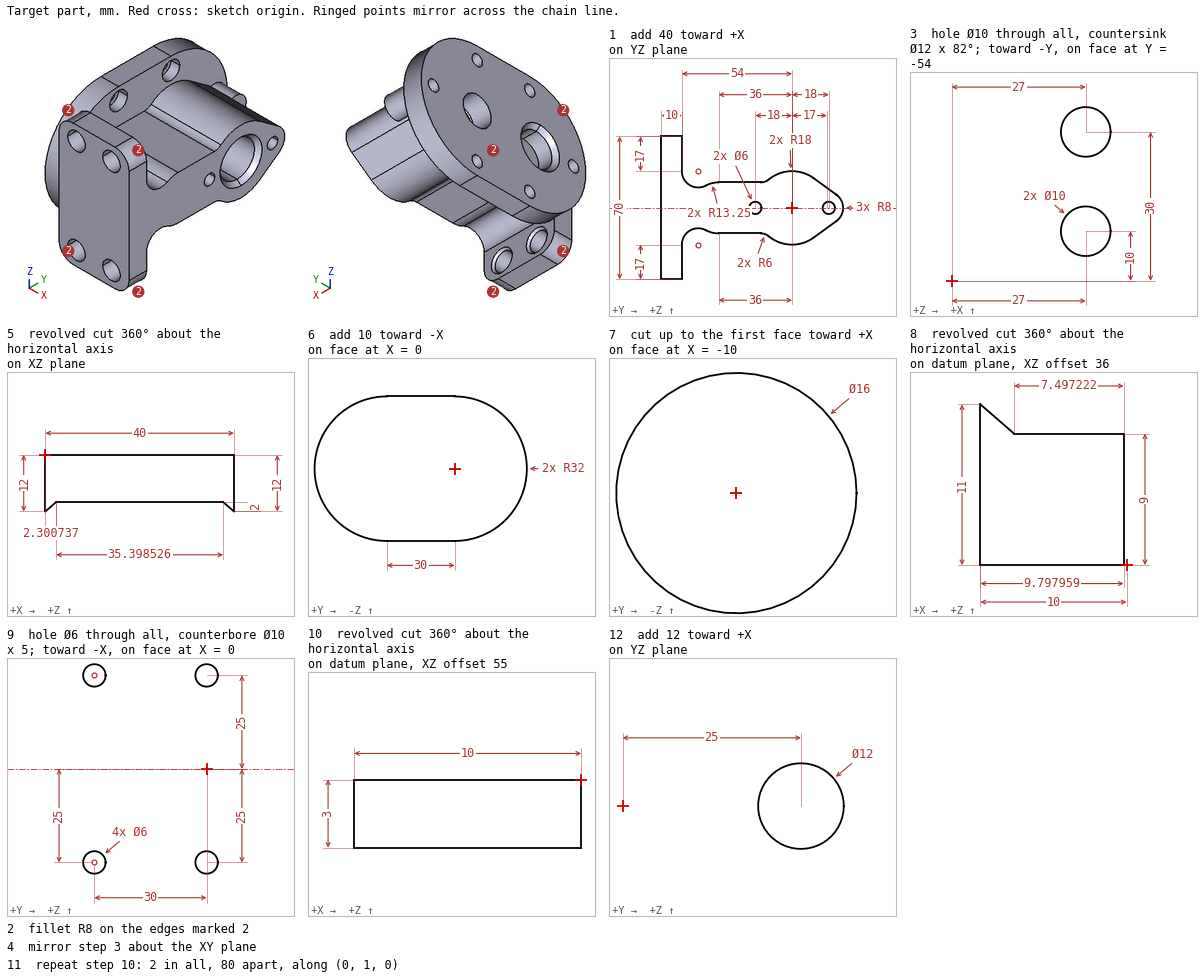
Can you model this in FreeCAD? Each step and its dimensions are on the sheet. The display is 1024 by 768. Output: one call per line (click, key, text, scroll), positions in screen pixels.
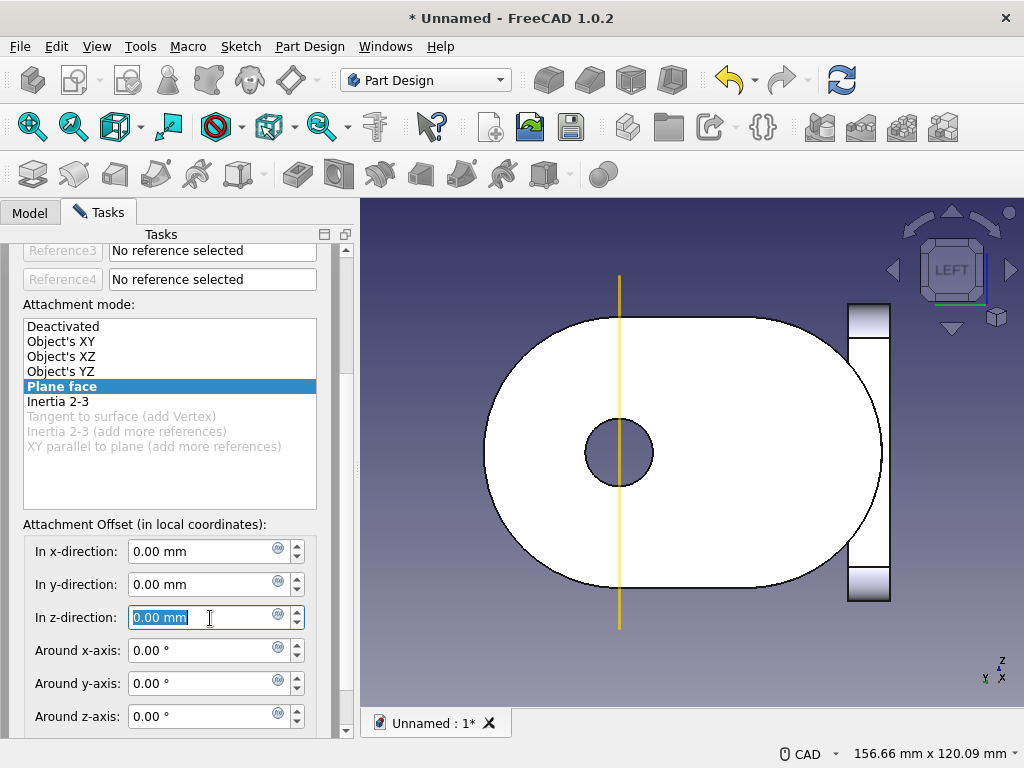
text(36)
key(Tab)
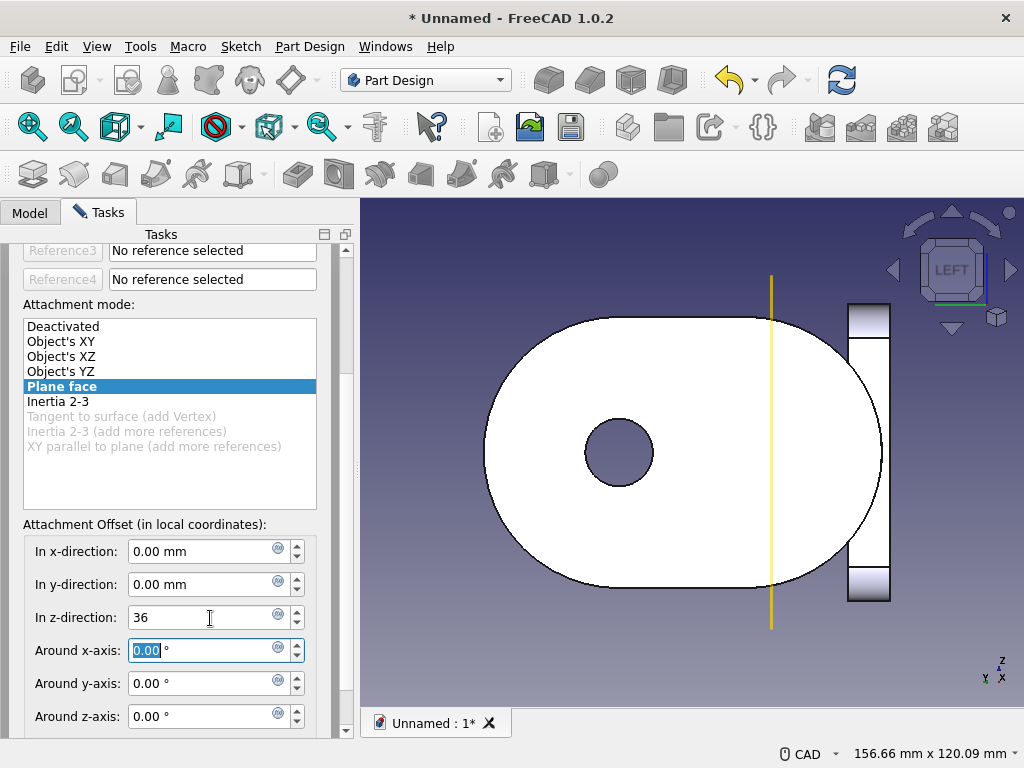
scroll(346, 491, up, 4)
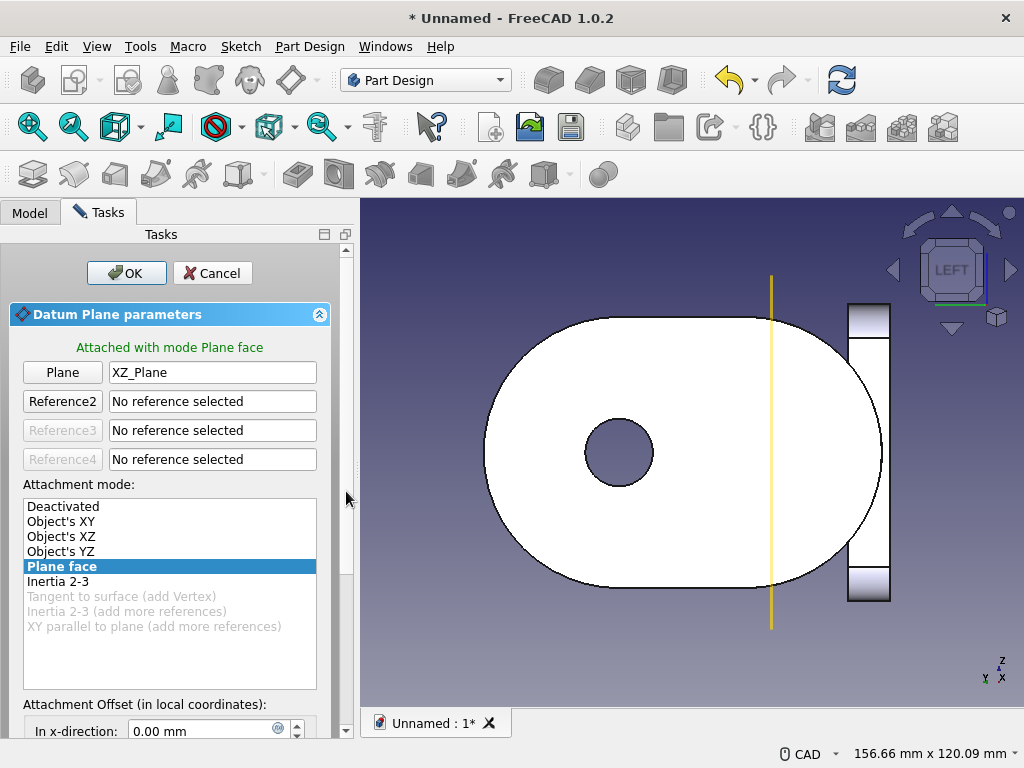
click(127, 273)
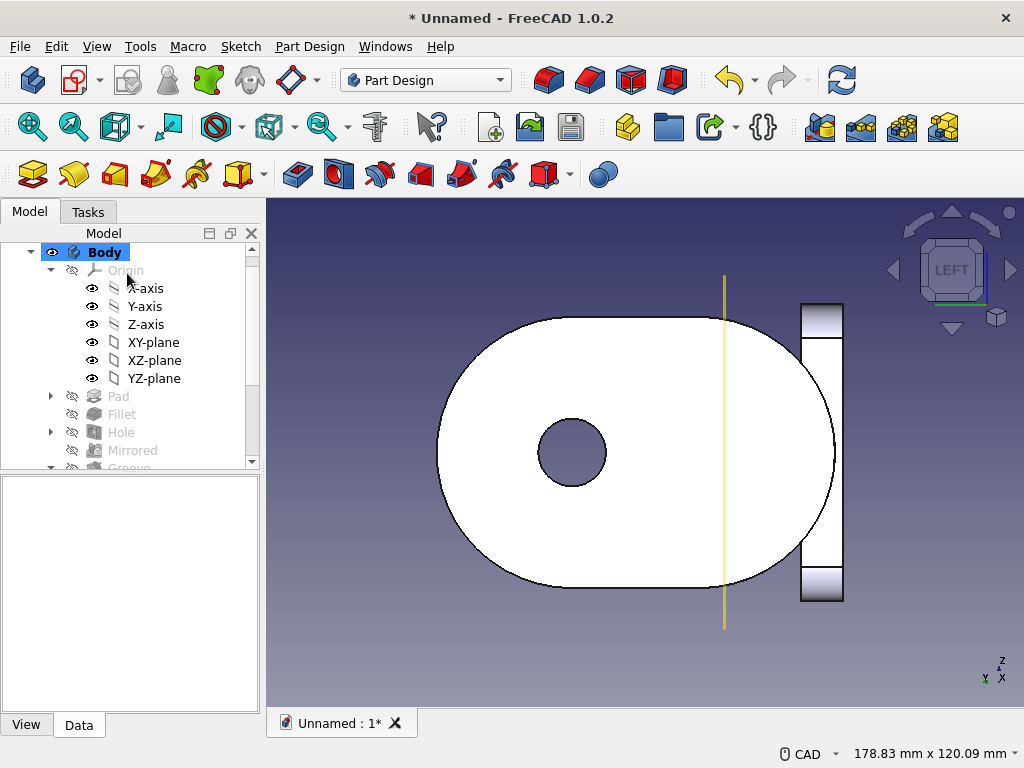
scroll(121, 356, down, 3)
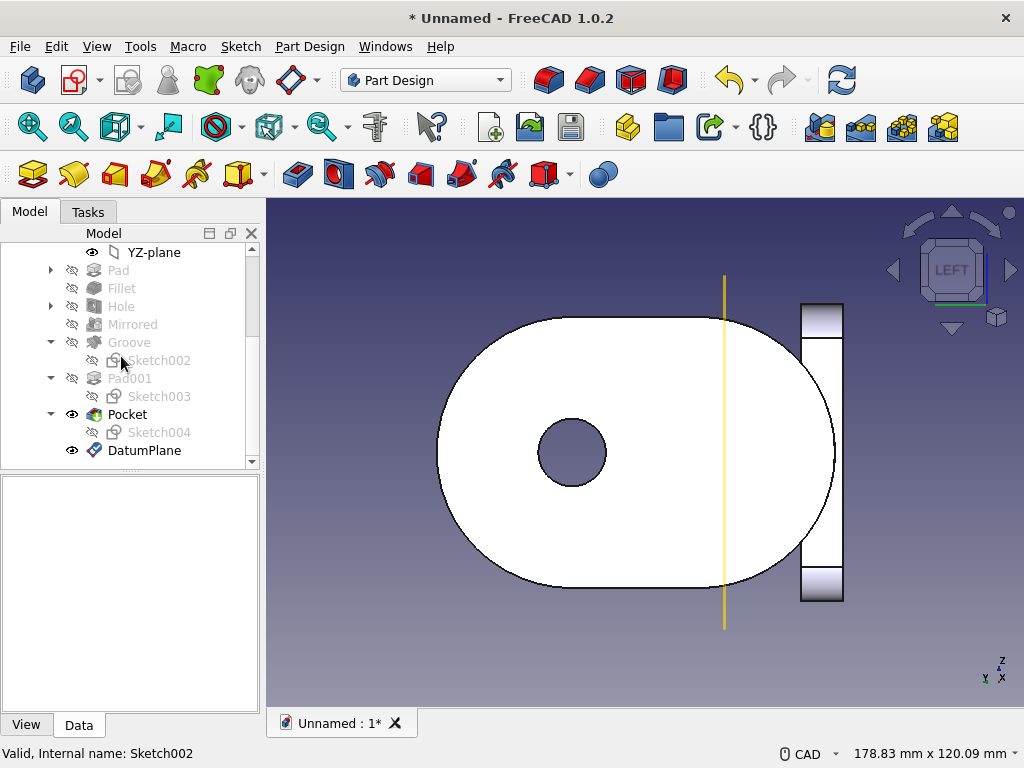
click(117, 450)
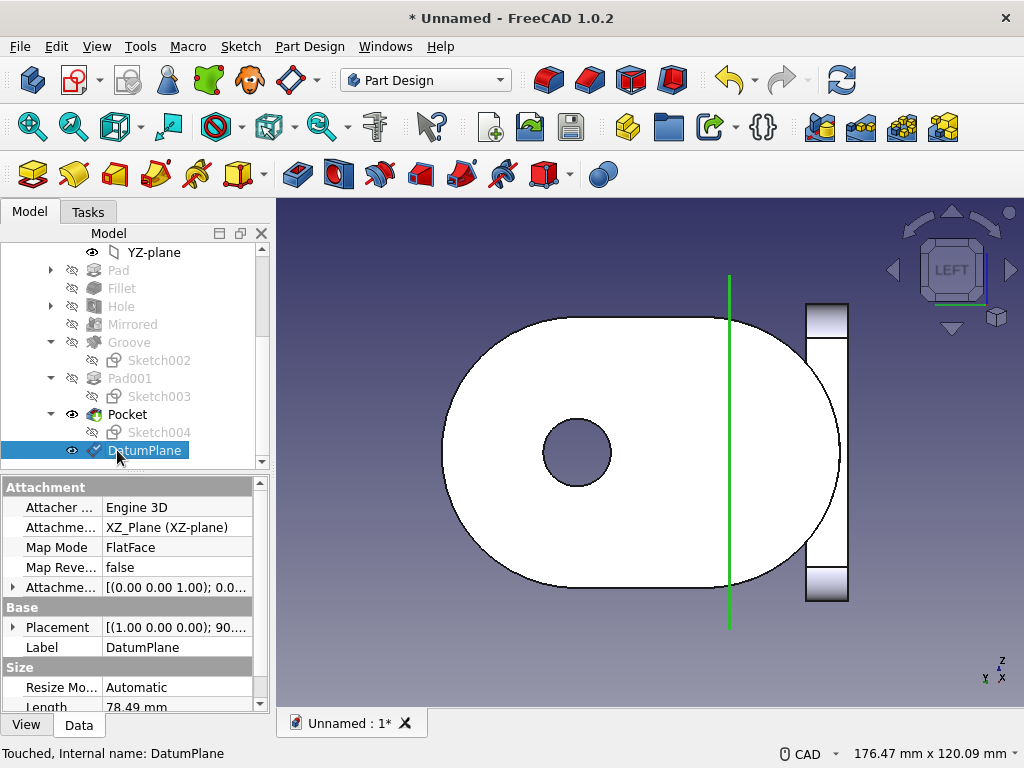
click(74, 80)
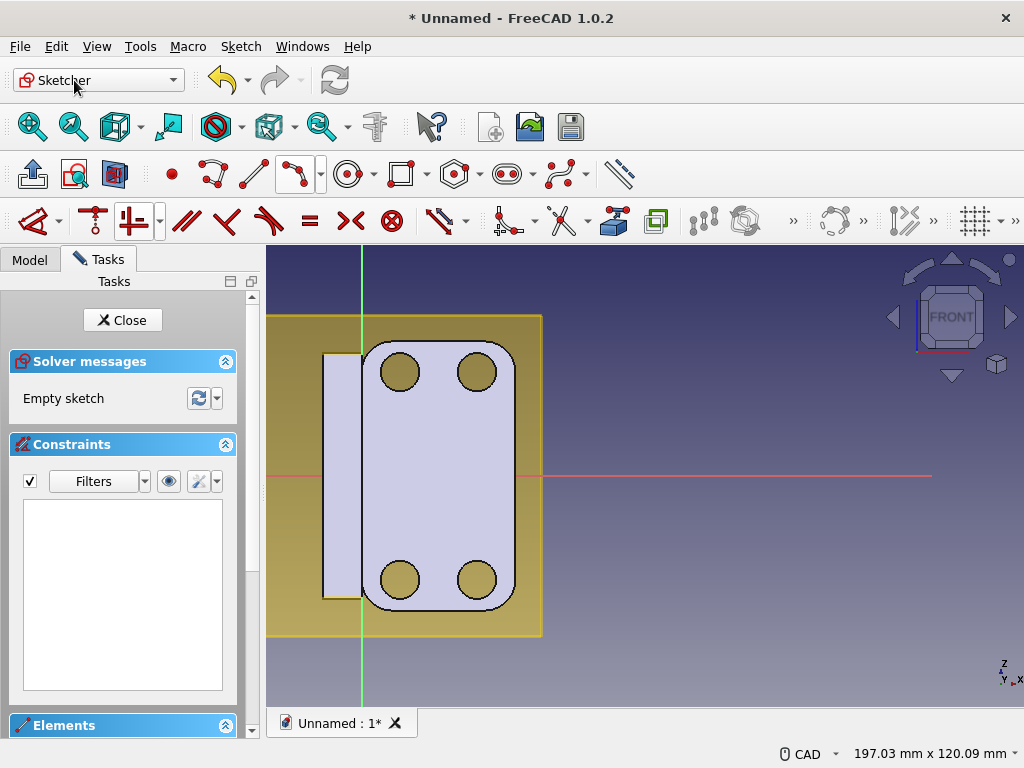
click(115, 174)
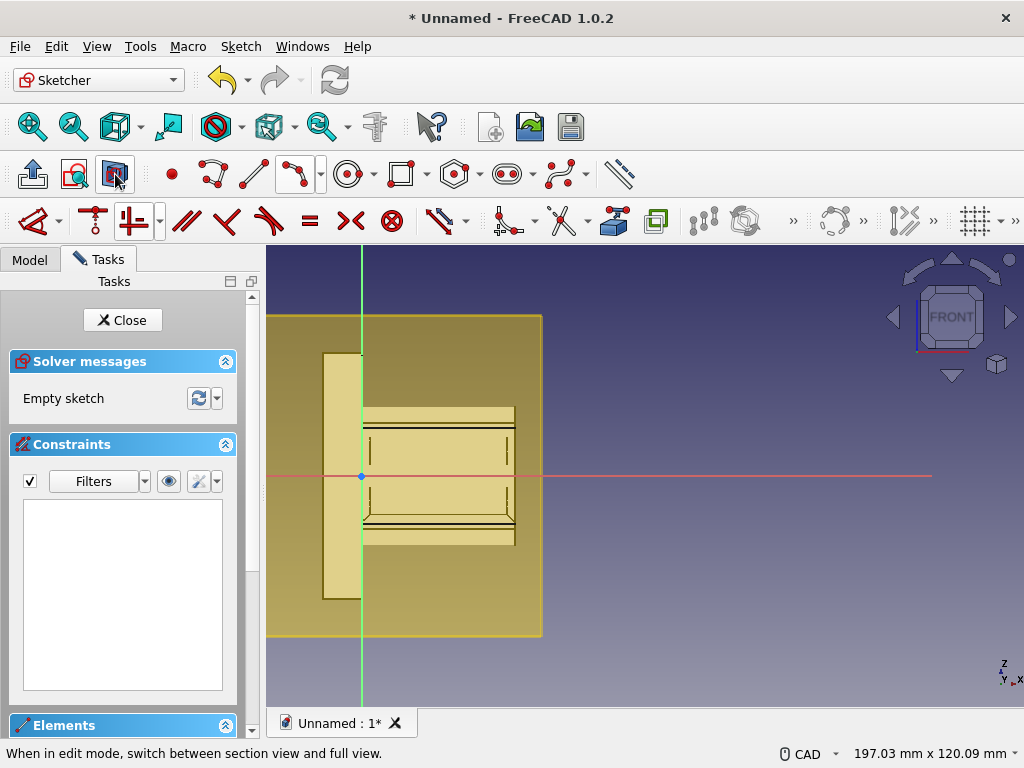
scroll(306, 452, up, 10)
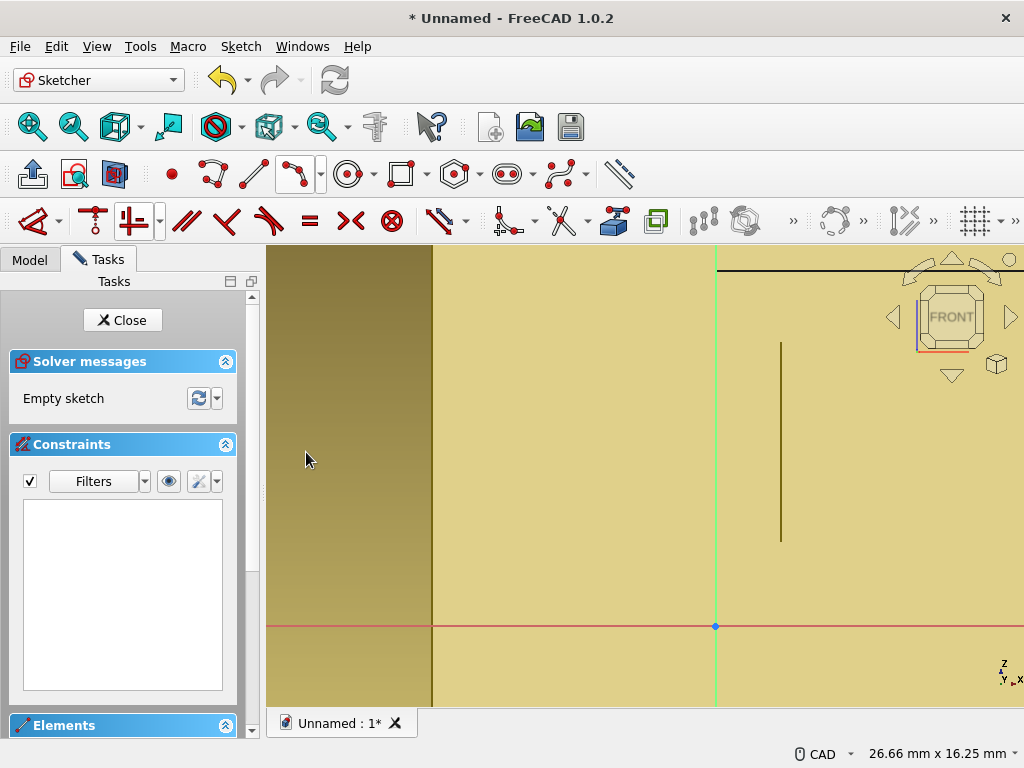
click(213, 174)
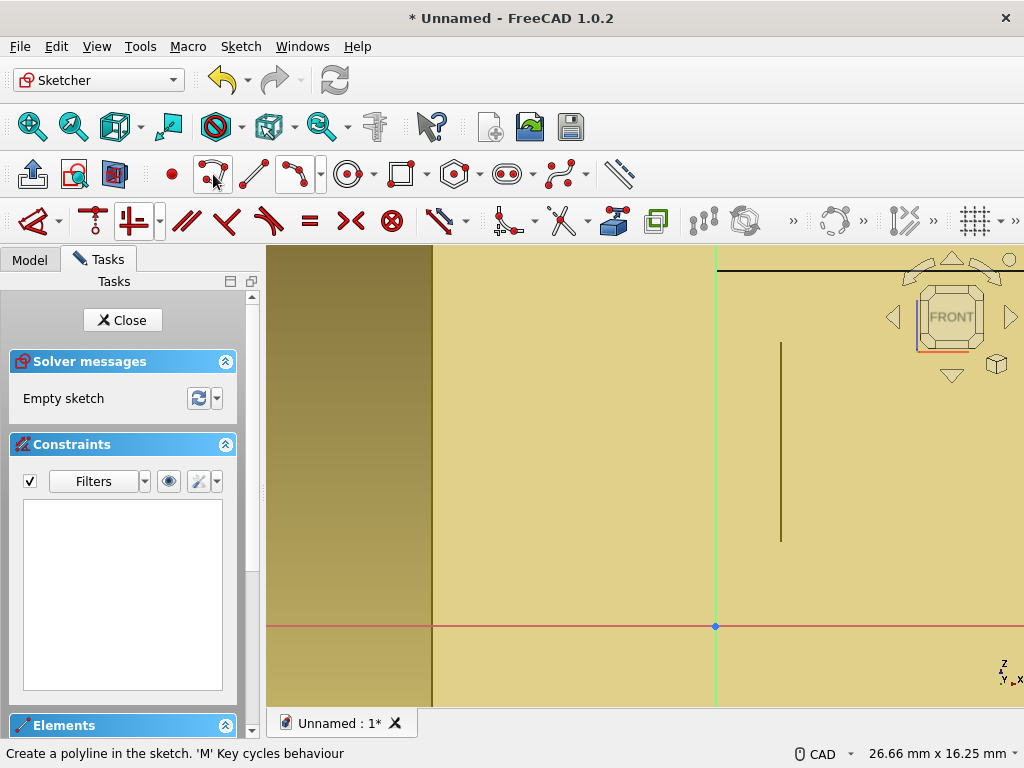
scroll(710, 626, up, 6)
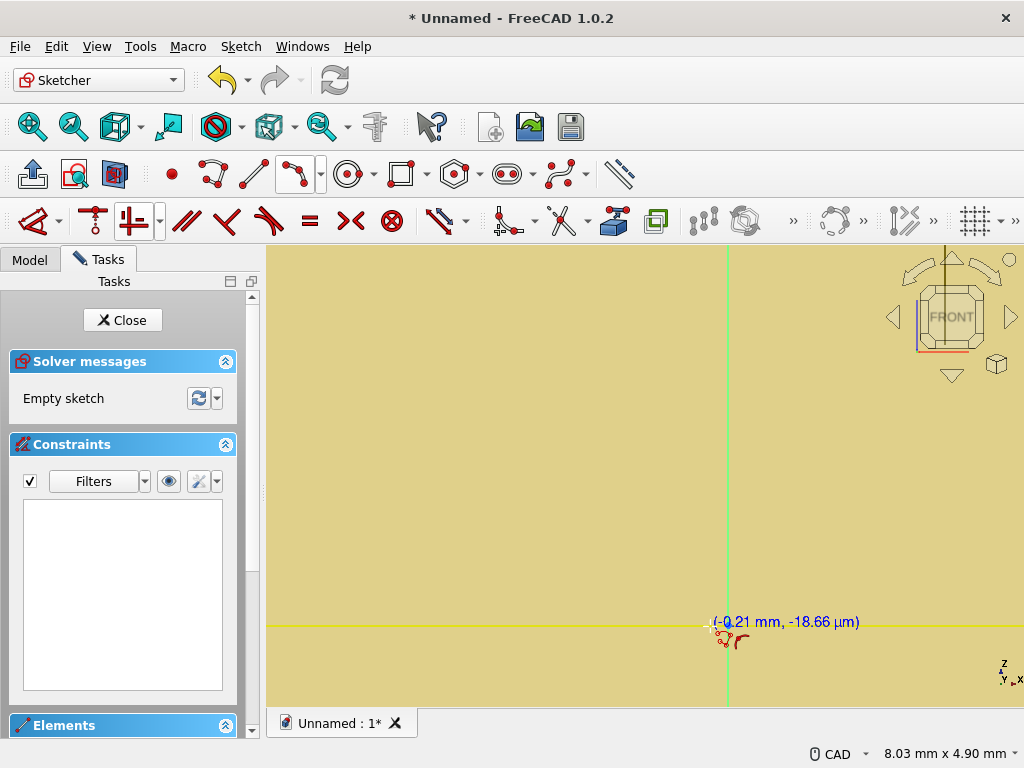
click(709, 626)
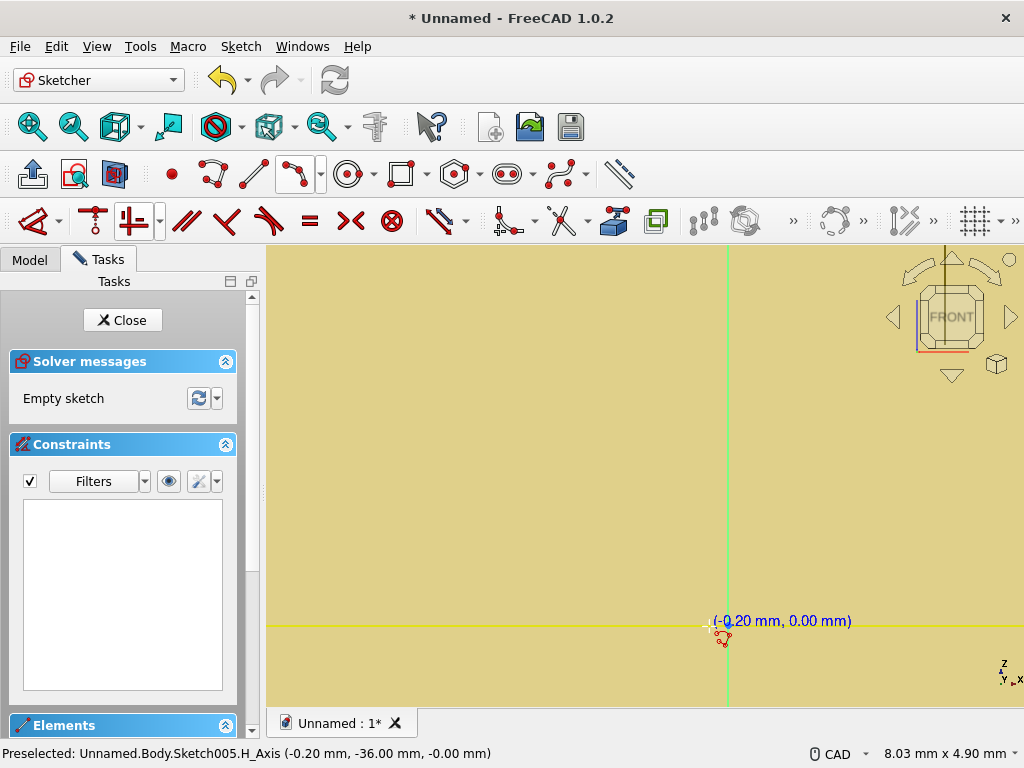
scroll(715, 635, down, 6)